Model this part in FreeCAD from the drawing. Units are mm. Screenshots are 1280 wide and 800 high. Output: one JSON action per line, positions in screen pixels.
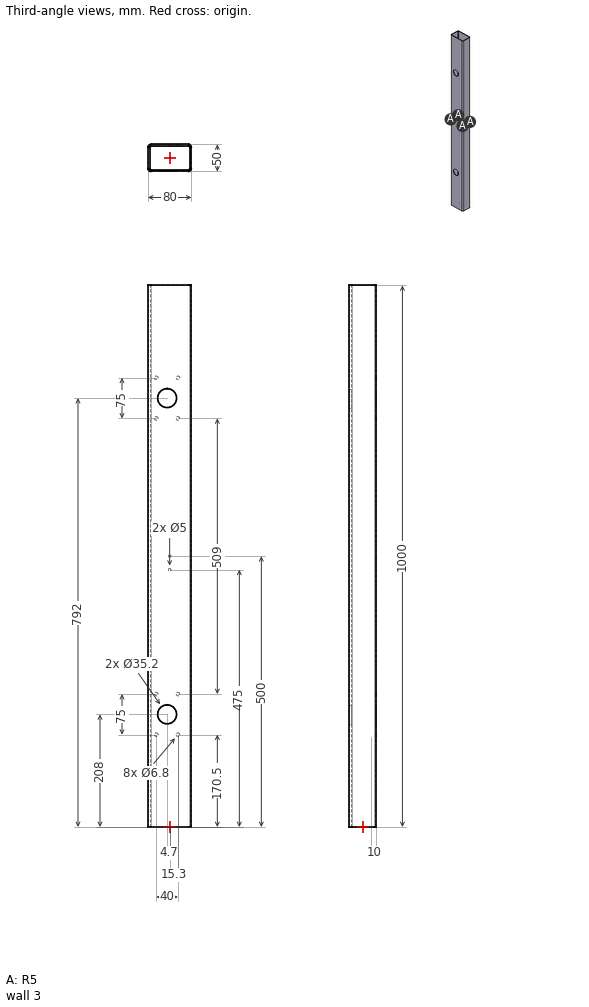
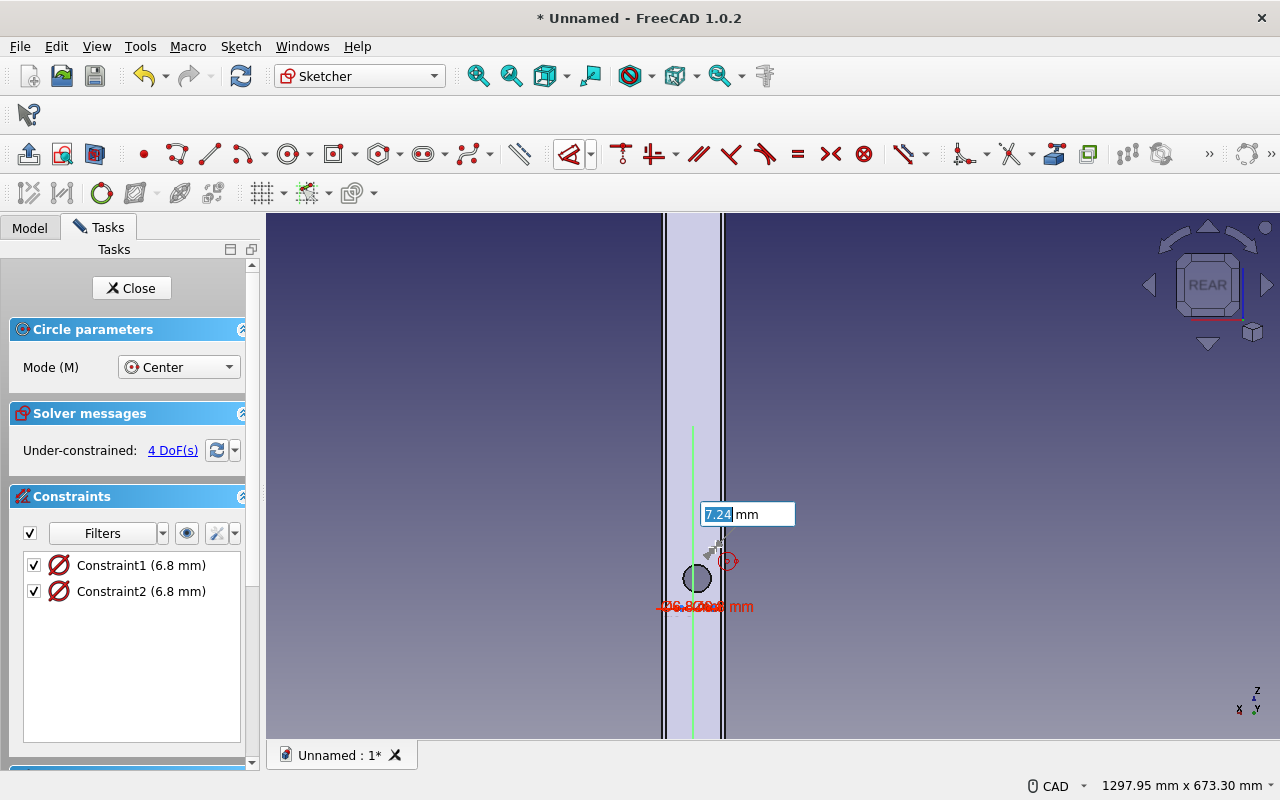
{"action": "type", "text": "6.8"}
{"action": "key", "text": "Return"}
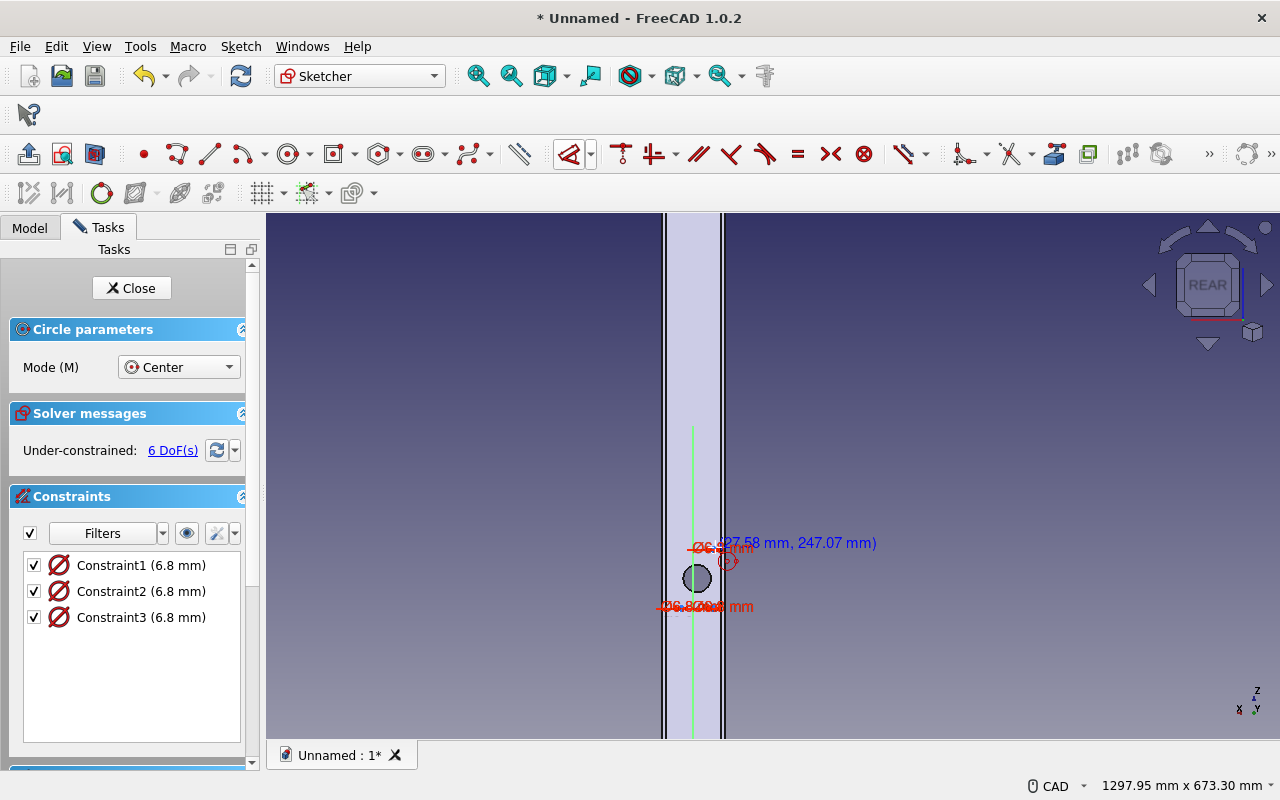
{"action": "scroll", "coordinate": [681, 549], "scroll_direction": "up", "scroll_amount": 11}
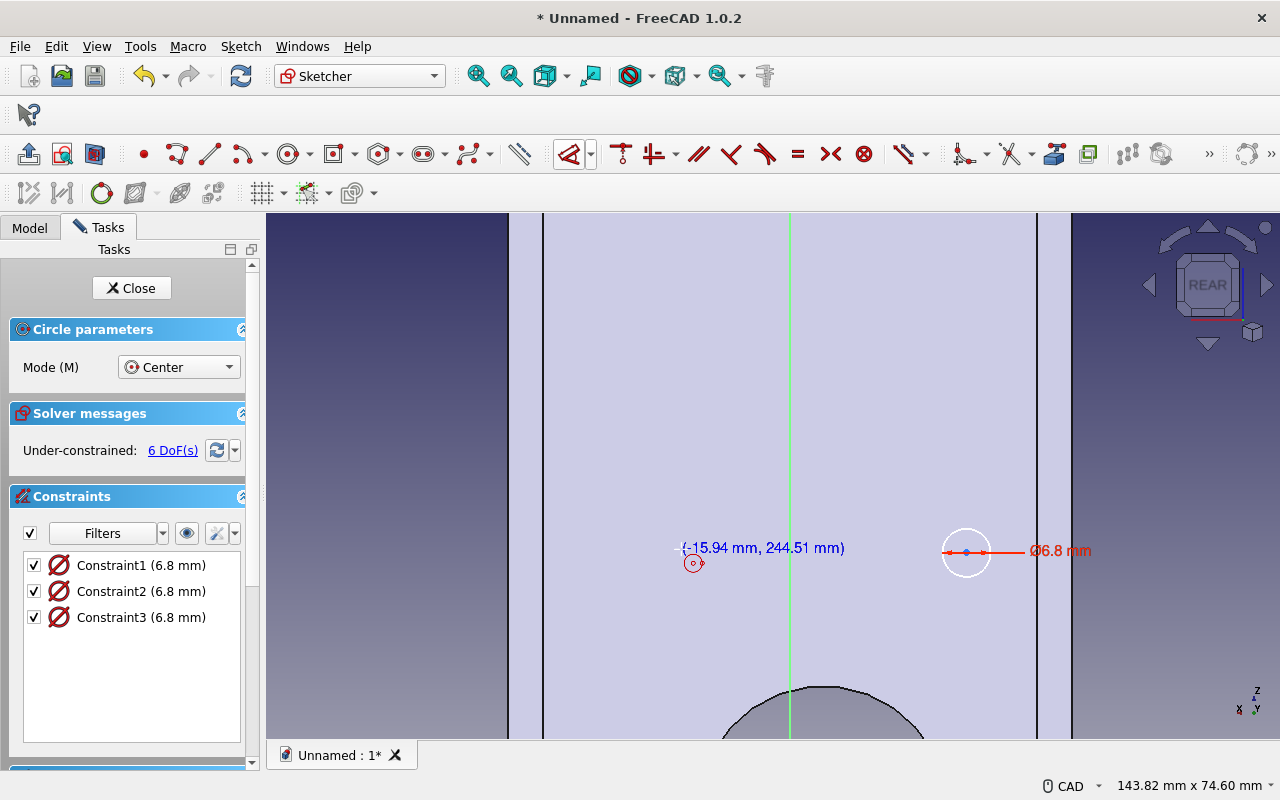
{"action": "scroll", "coordinate": [697, 550], "scroll_direction": "down", "scroll_amount": 14}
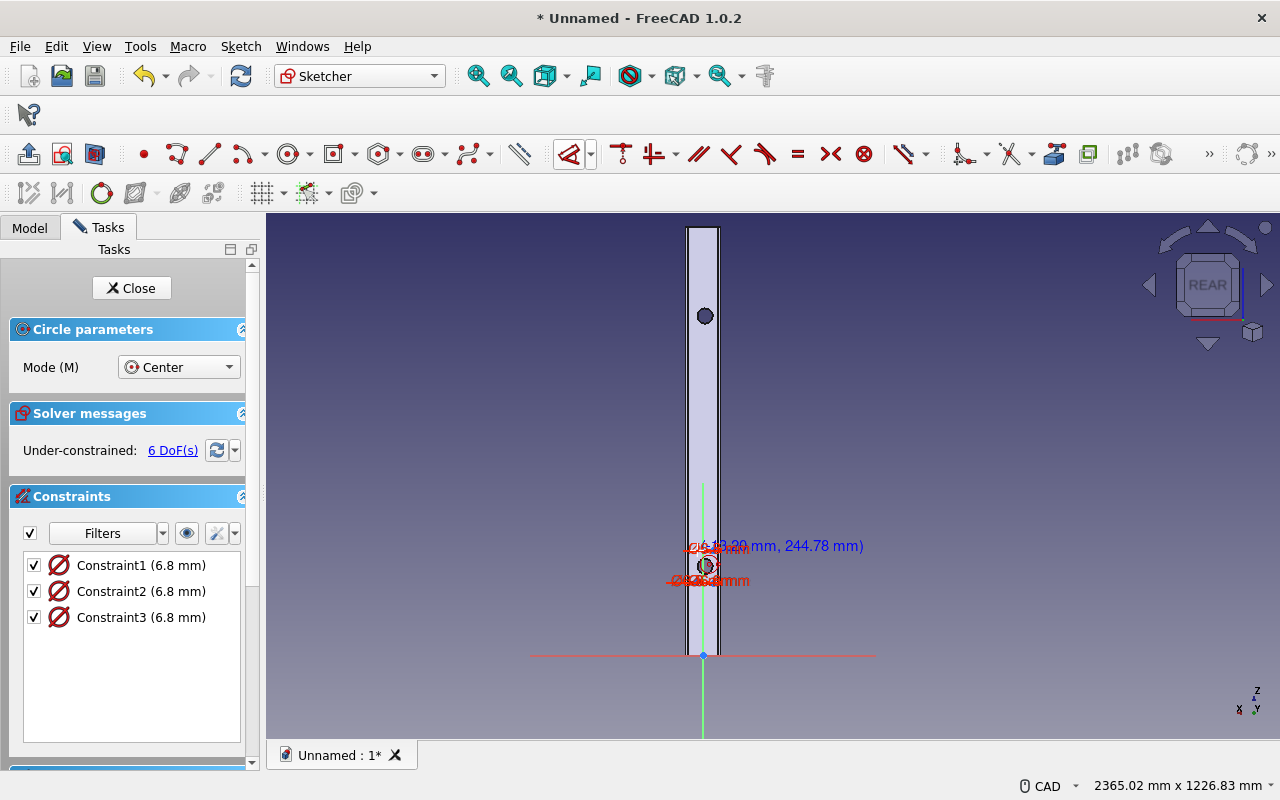
{"action": "scroll", "coordinate": [696, 550], "scroll_direction": "up", "scroll_amount": 5}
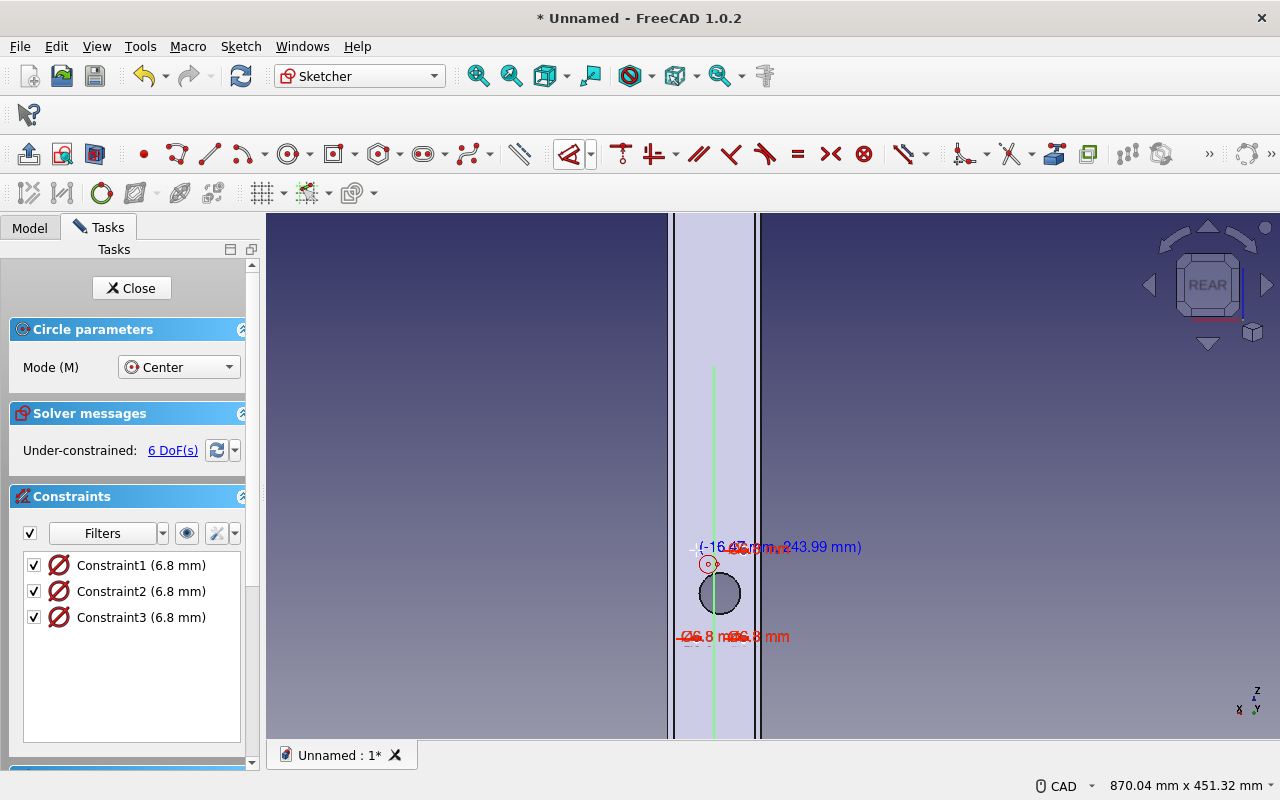
{"action": "left_click", "coordinate": [697, 550]}
{"action": "mouse_move", "coordinate": [699, 547]}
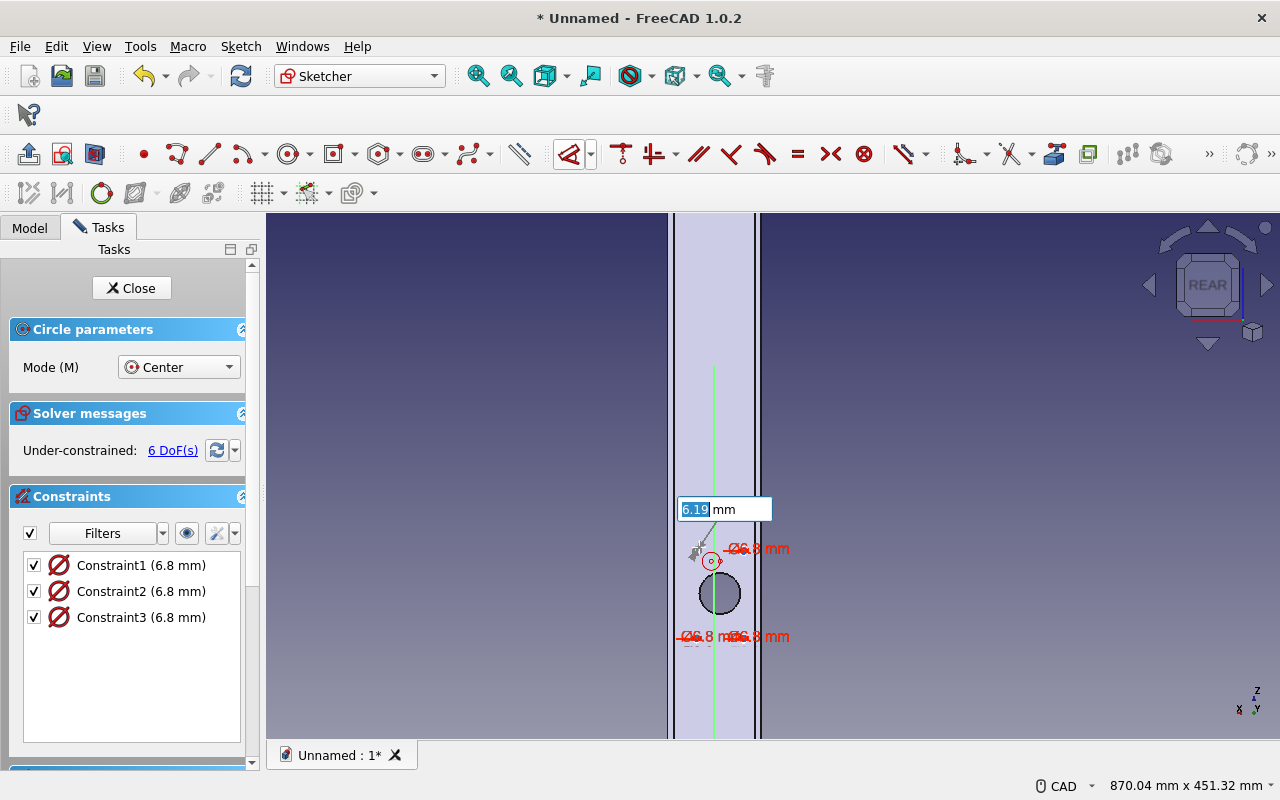
{"action": "type", "text": "6.8"}
{"action": "key", "text": "Return"}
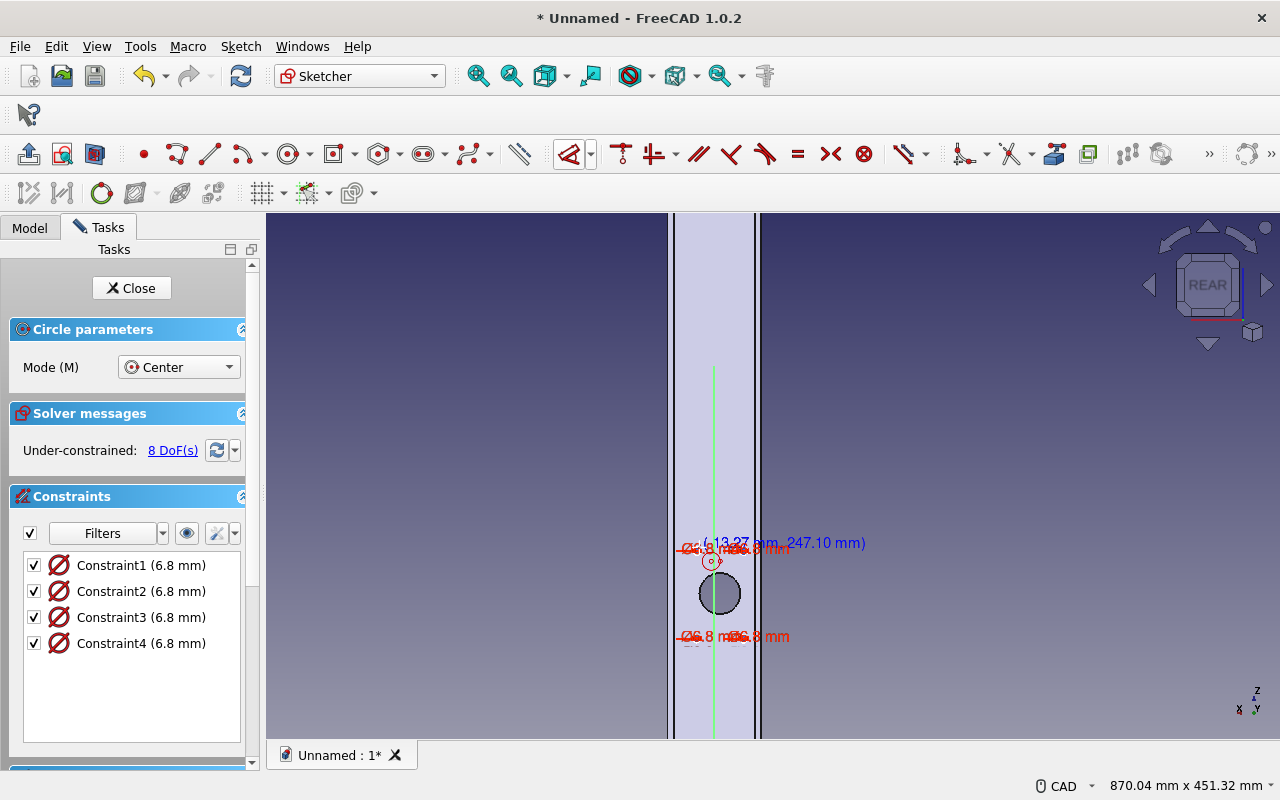
{"action": "scroll", "coordinate": [696, 549], "scroll_direction": "down", "scroll_amount": 5}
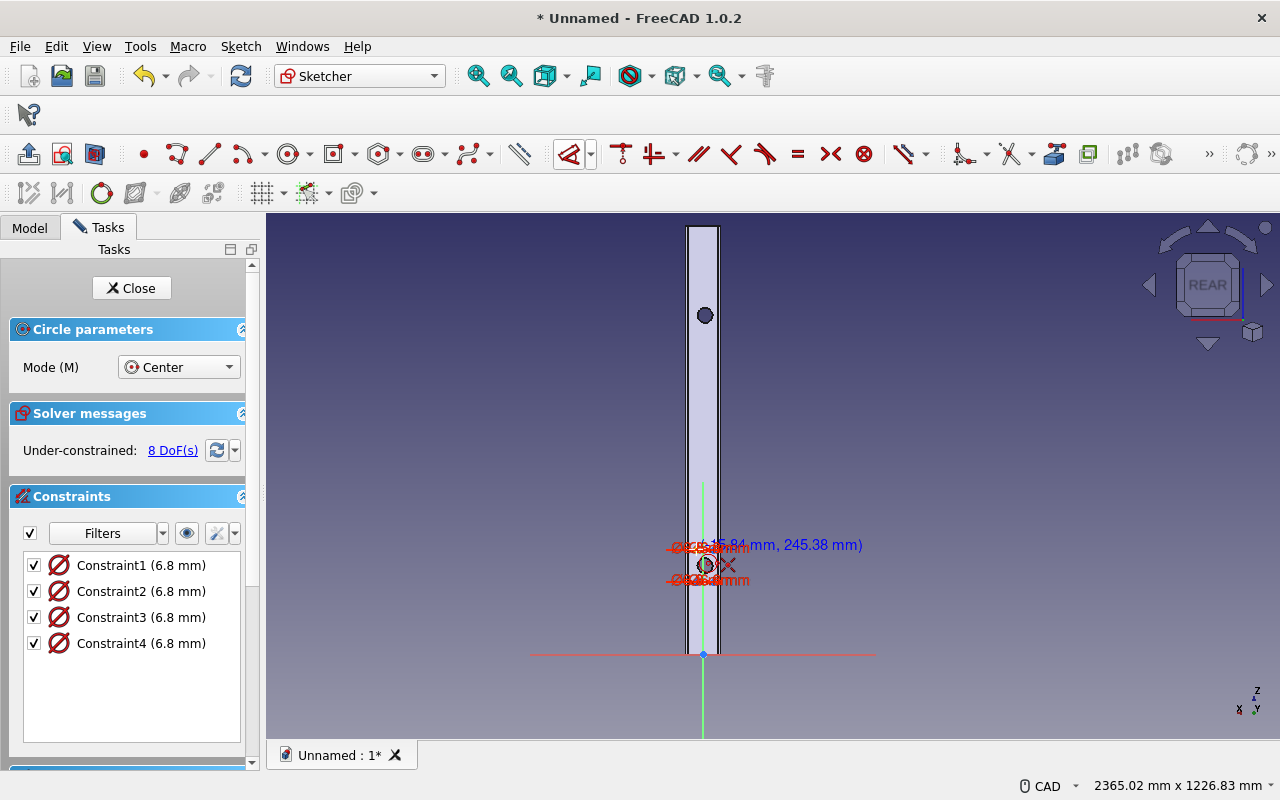
{"action": "scroll", "coordinate": [696, 331], "scroll_direction": "up", "scroll_amount": 14}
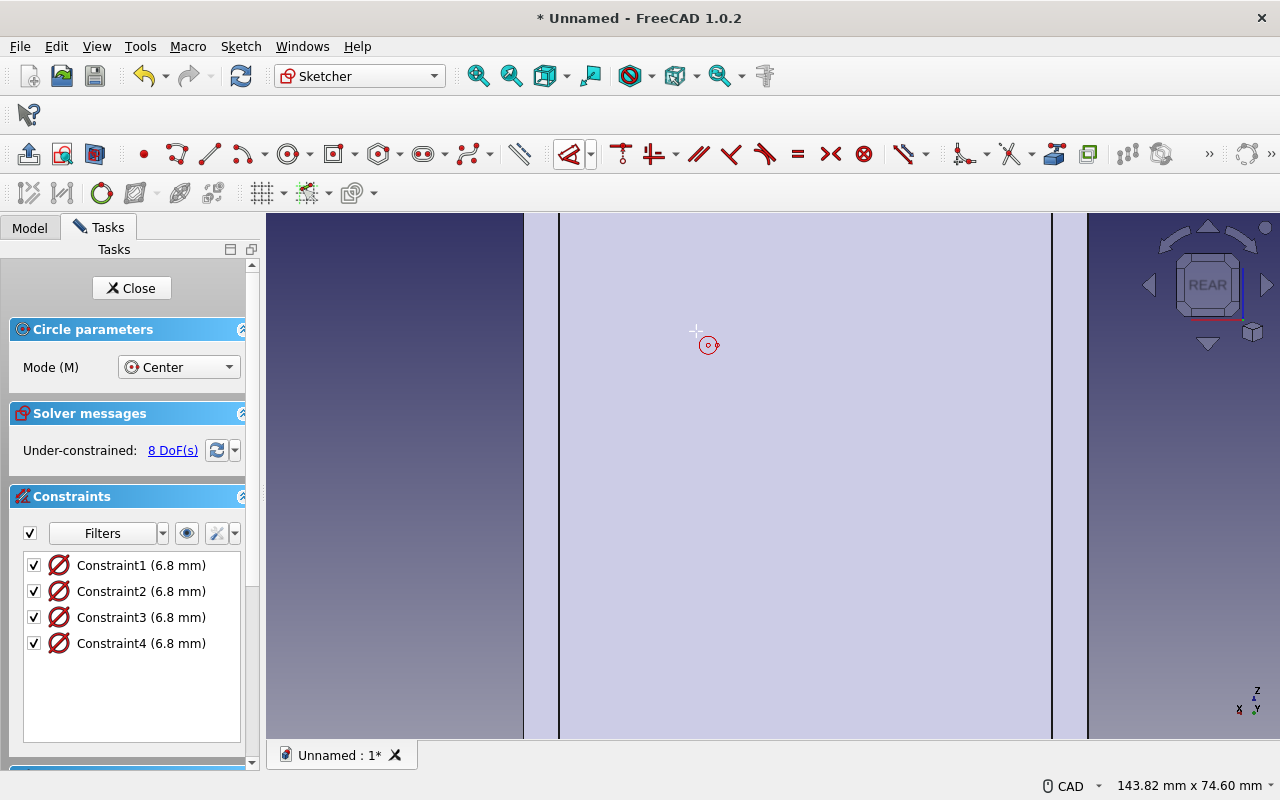
{"action": "scroll", "coordinate": [696, 331], "scroll_direction": "down", "scroll_amount": 14}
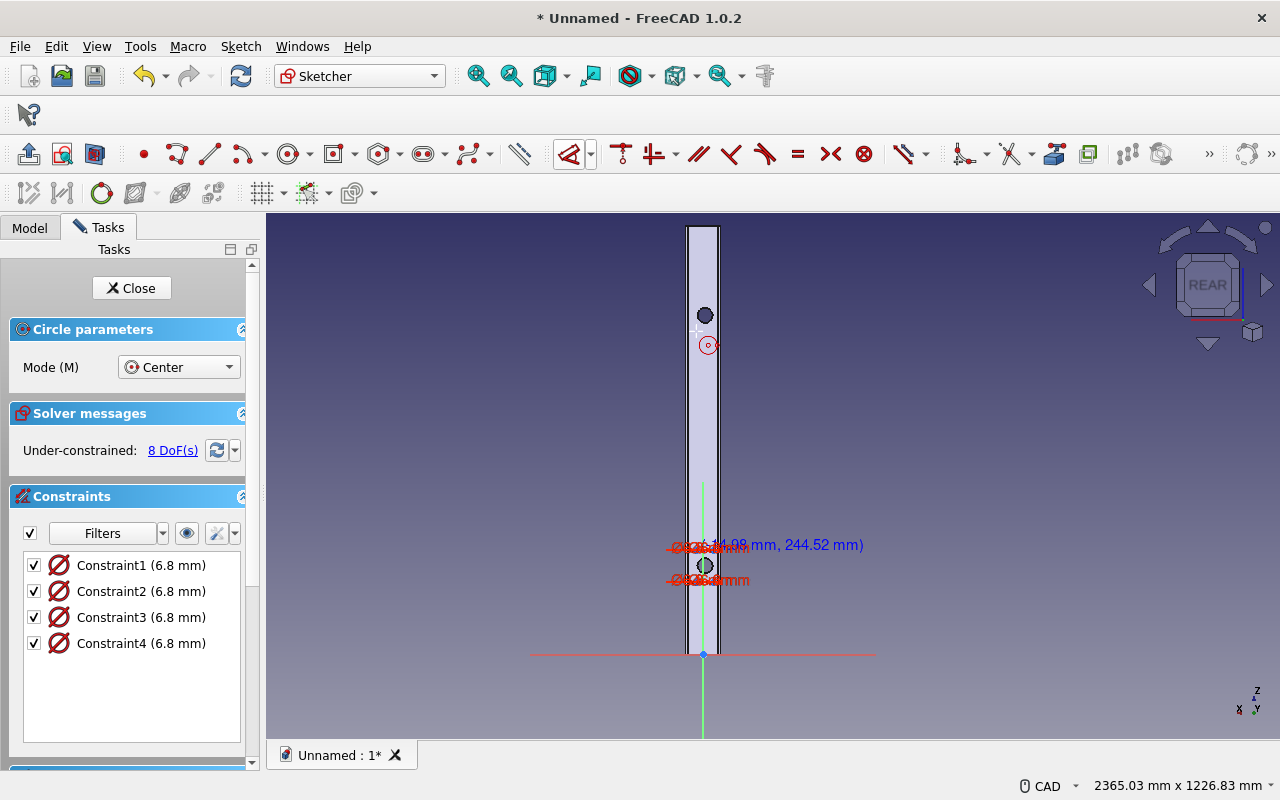
{"action": "scroll", "coordinate": [696, 331], "scroll_direction": "up", "scroll_amount": 5}